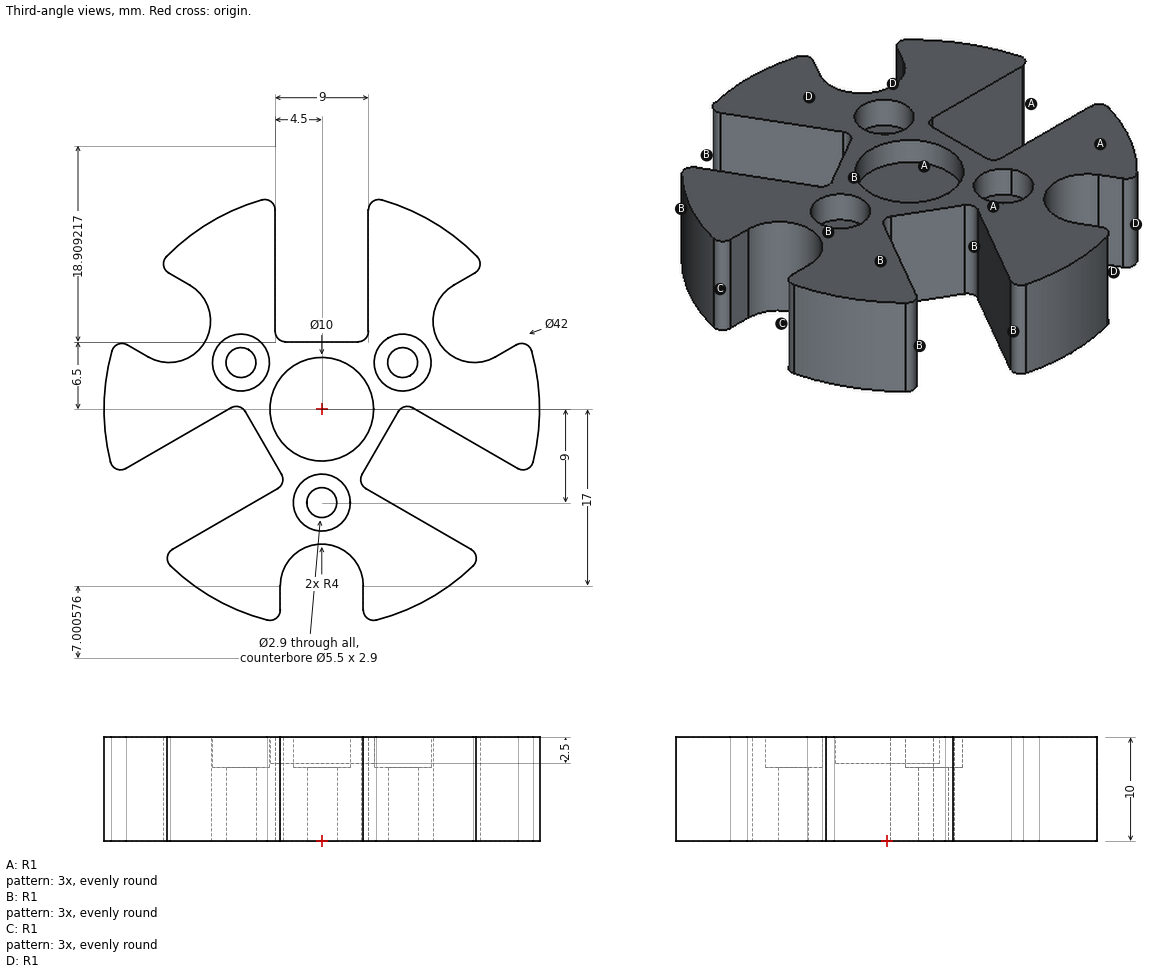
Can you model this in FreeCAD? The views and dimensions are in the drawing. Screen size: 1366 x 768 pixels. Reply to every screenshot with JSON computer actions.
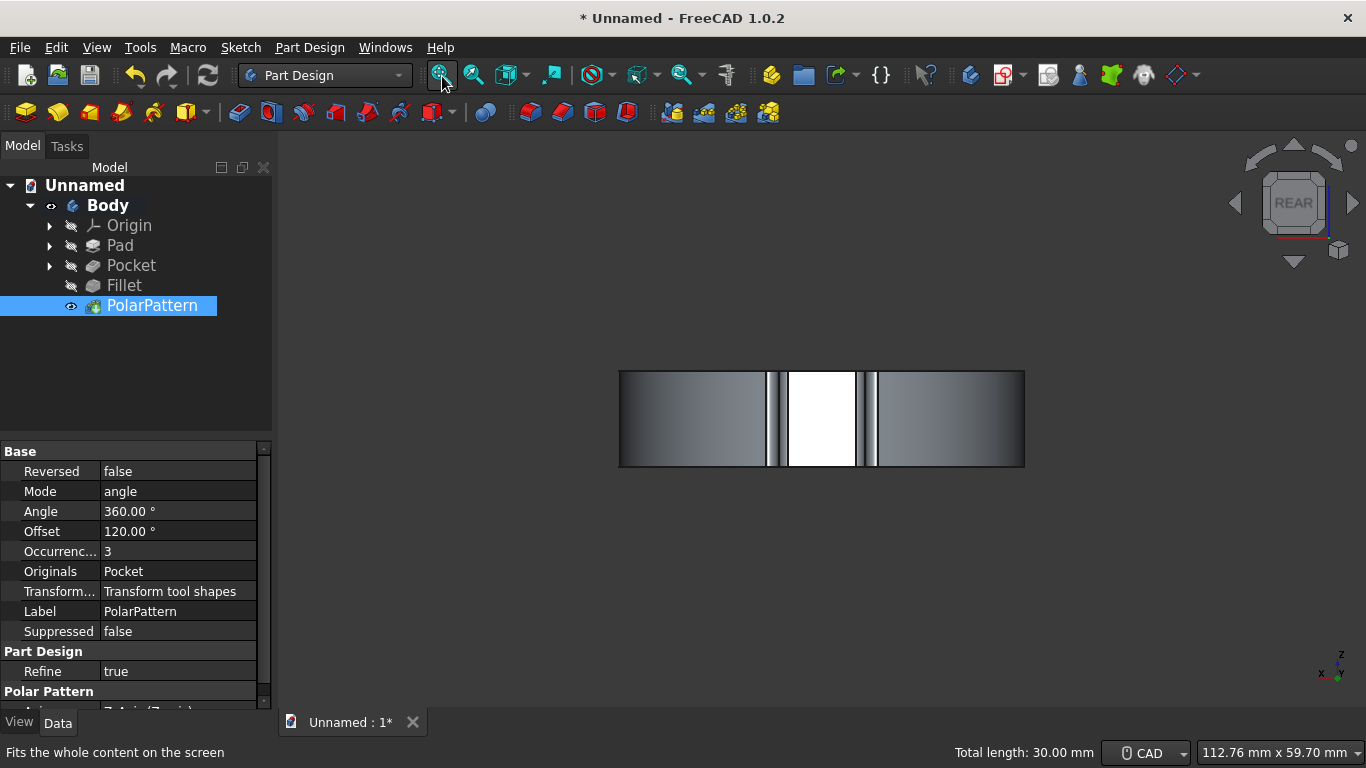
{"action": "left_click", "coordinate": [442, 76]}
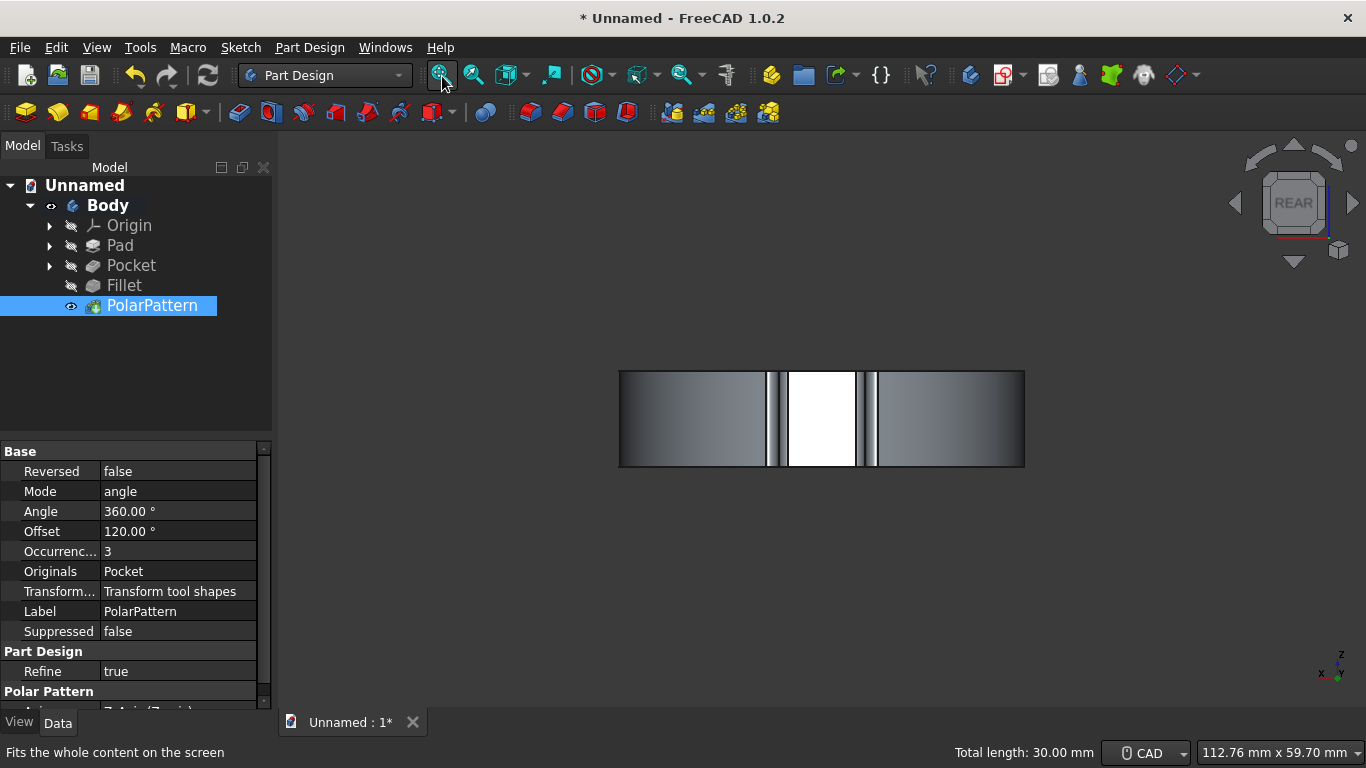
{"action": "key", "text": "6"}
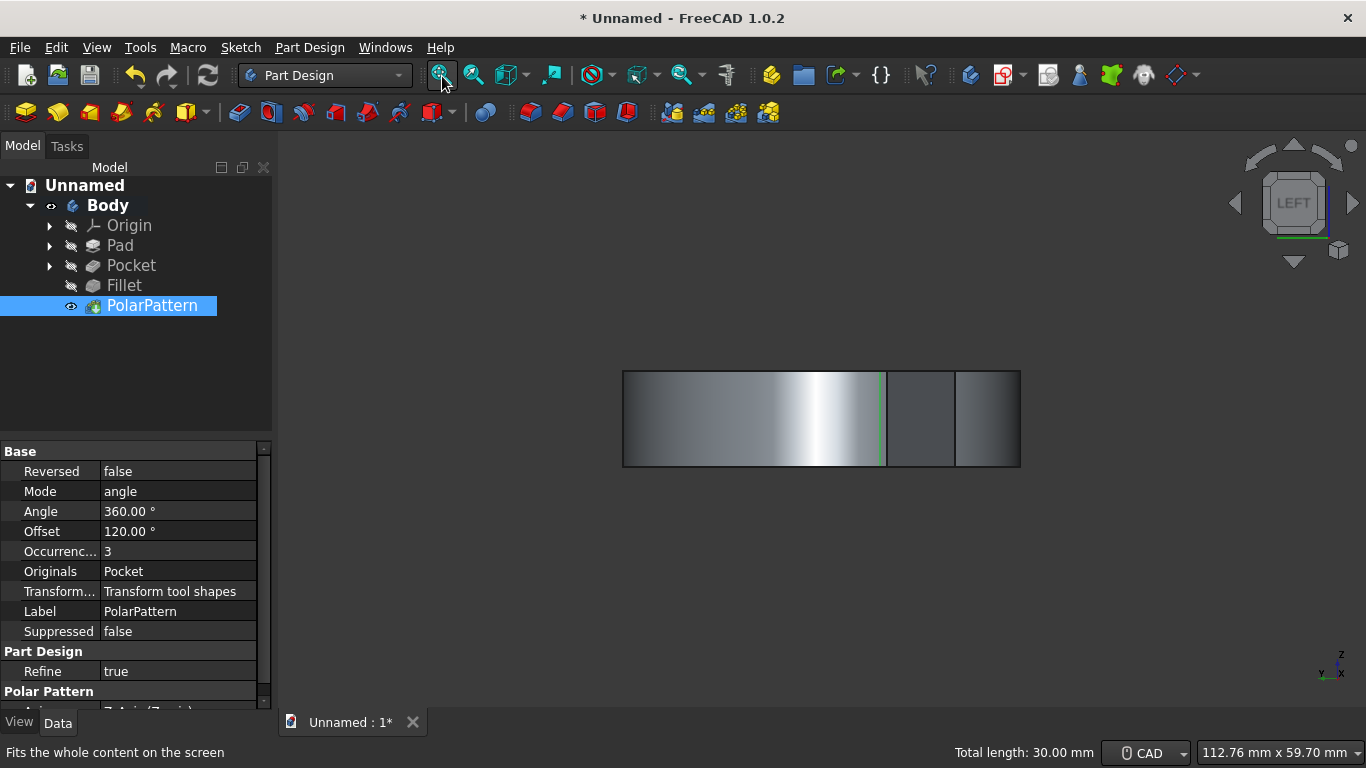
{"action": "left_click", "coordinate": [442, 76]}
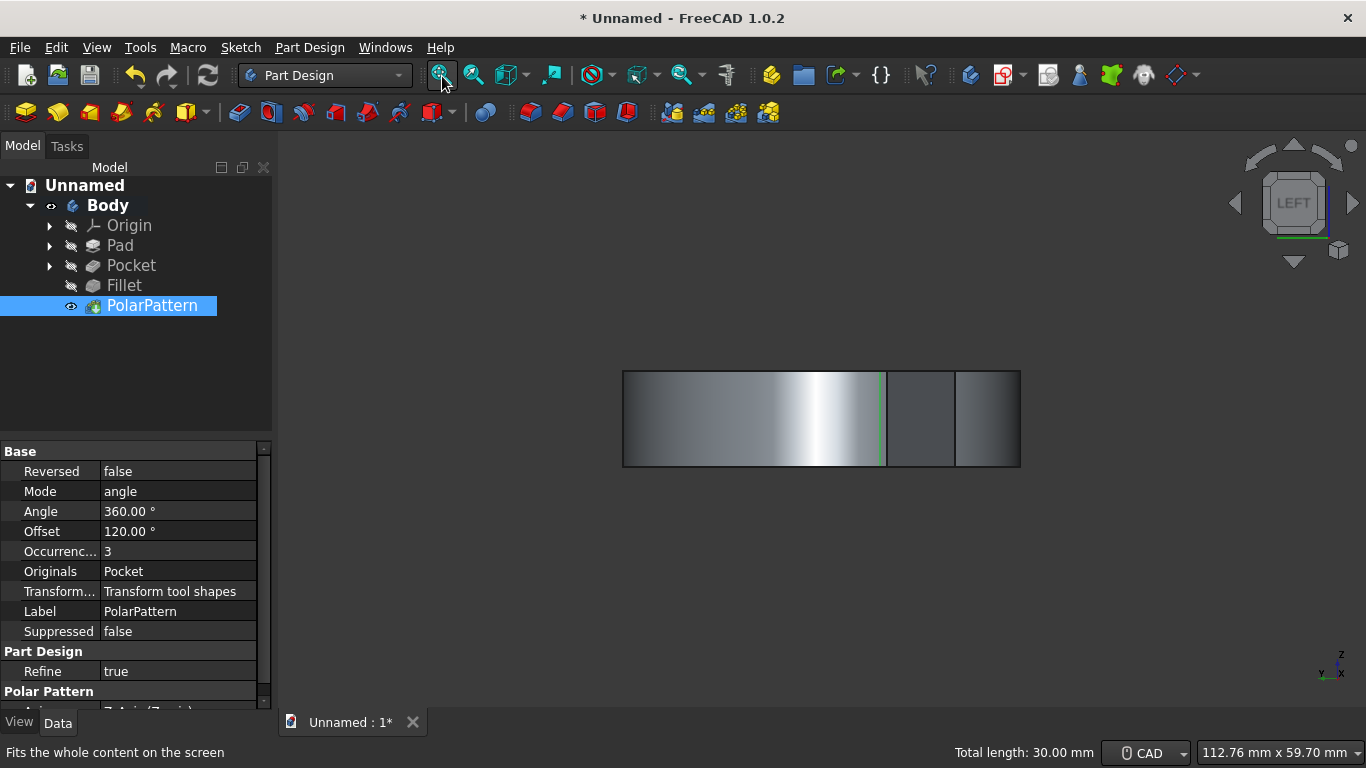
{"action": "left_click", "coordinate": [955, 418], "text": "ctrl"}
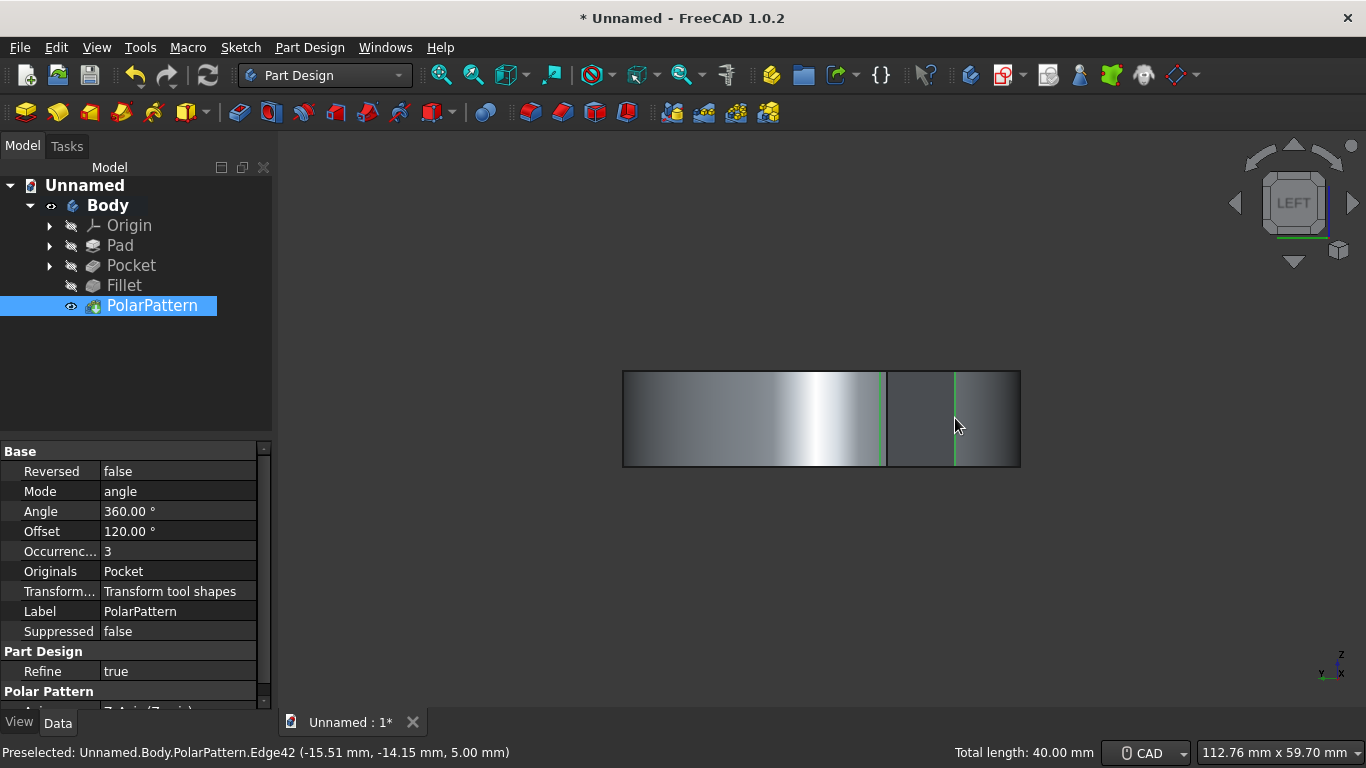
{"action": "key", "text": "v 3"}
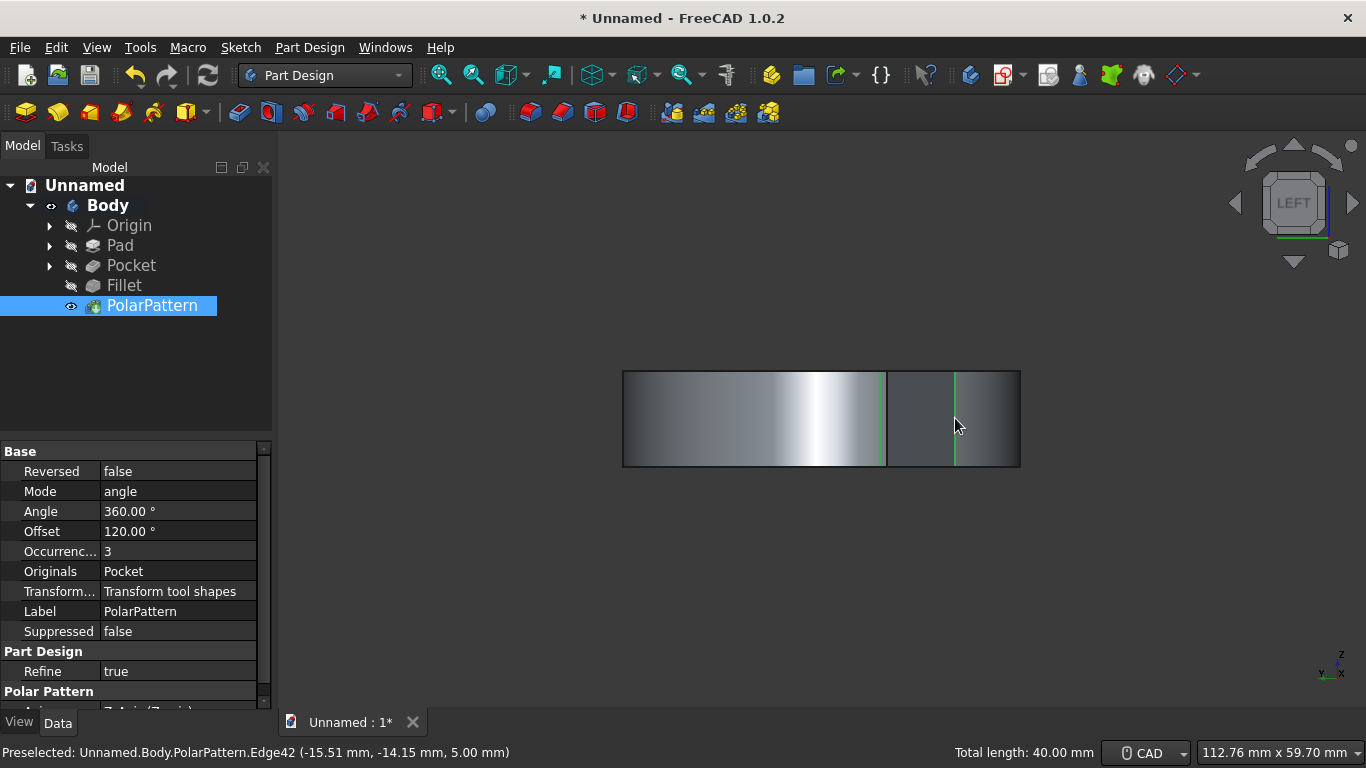
{"action": "key", "text": "0"}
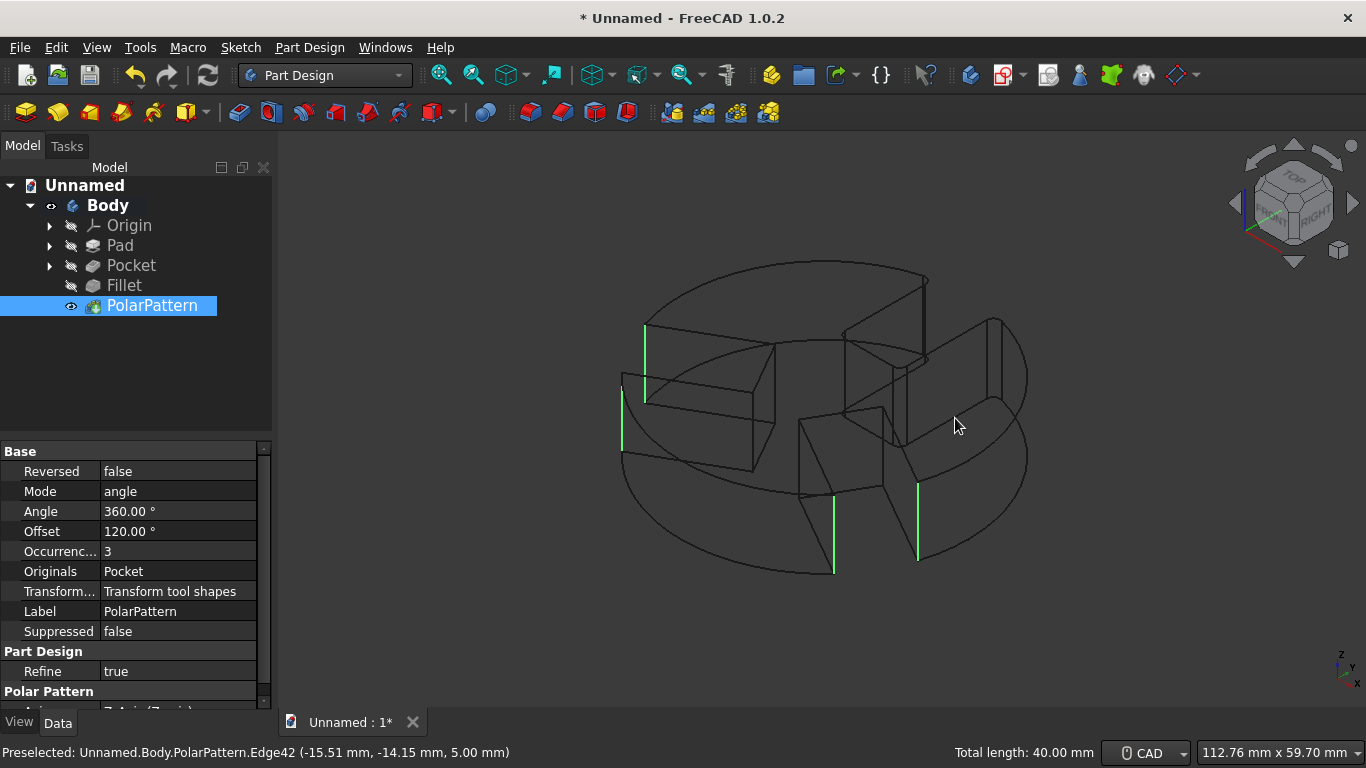
{"action": "left_click", "coordinate": [753, 431], "text": "ctrl"}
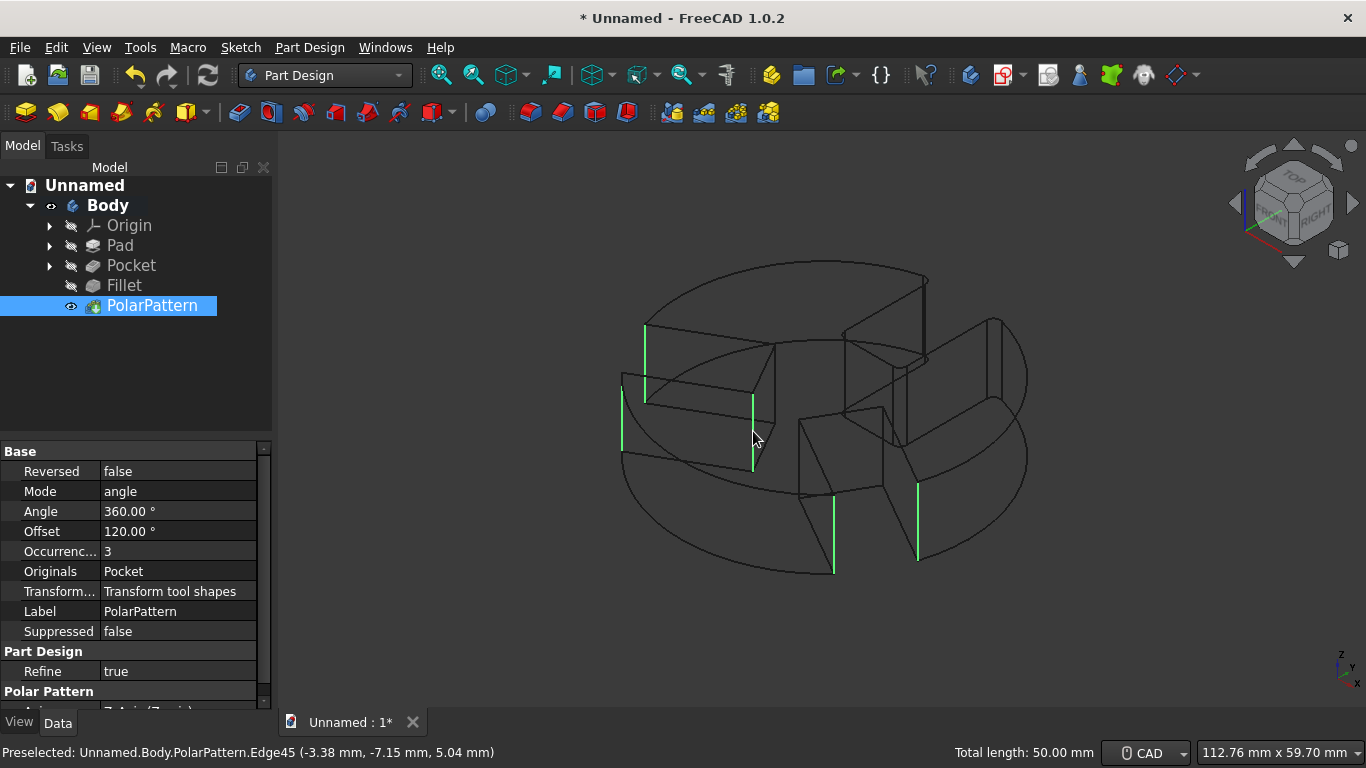
{"action": "left_click", "coordinate": [775, 383], "text": "ctrl"}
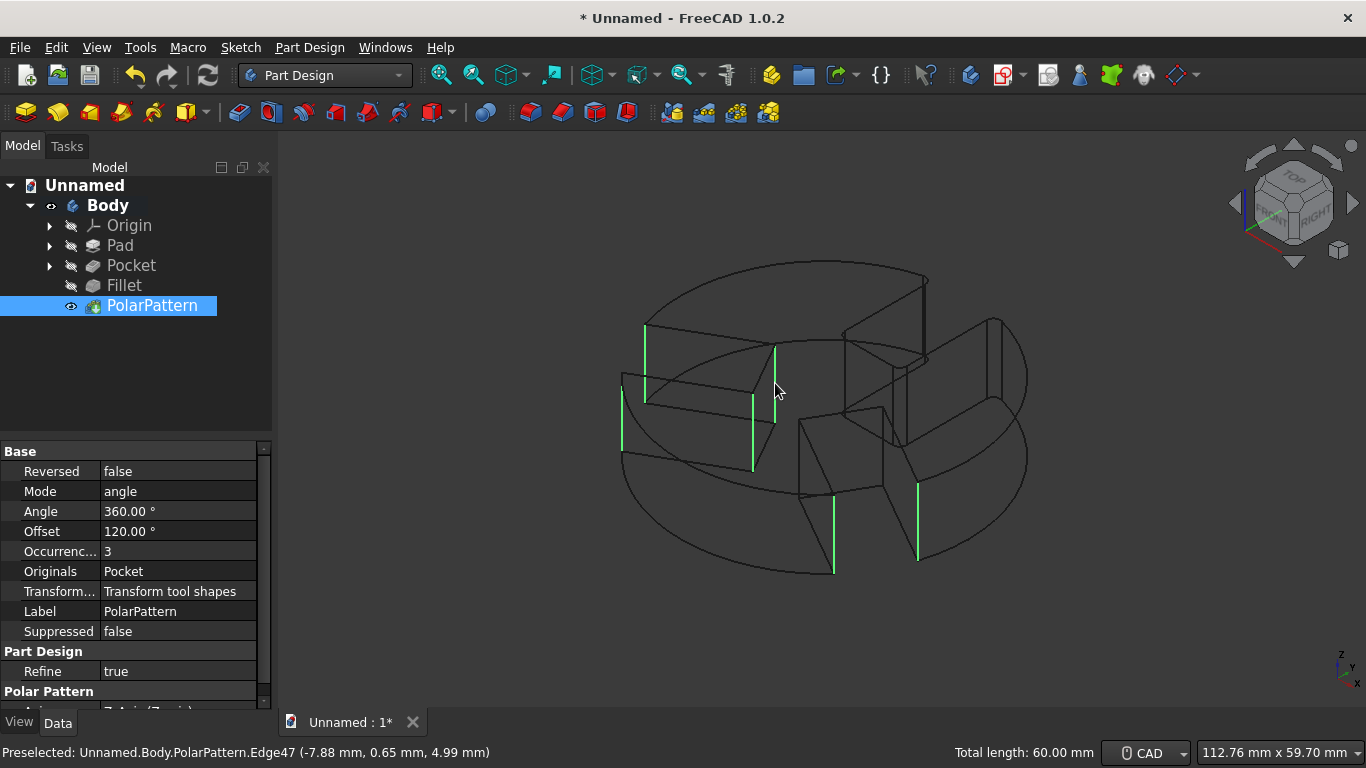
{"action": "left_click", "coordinate": [883, 445], "text": "ctrl"}